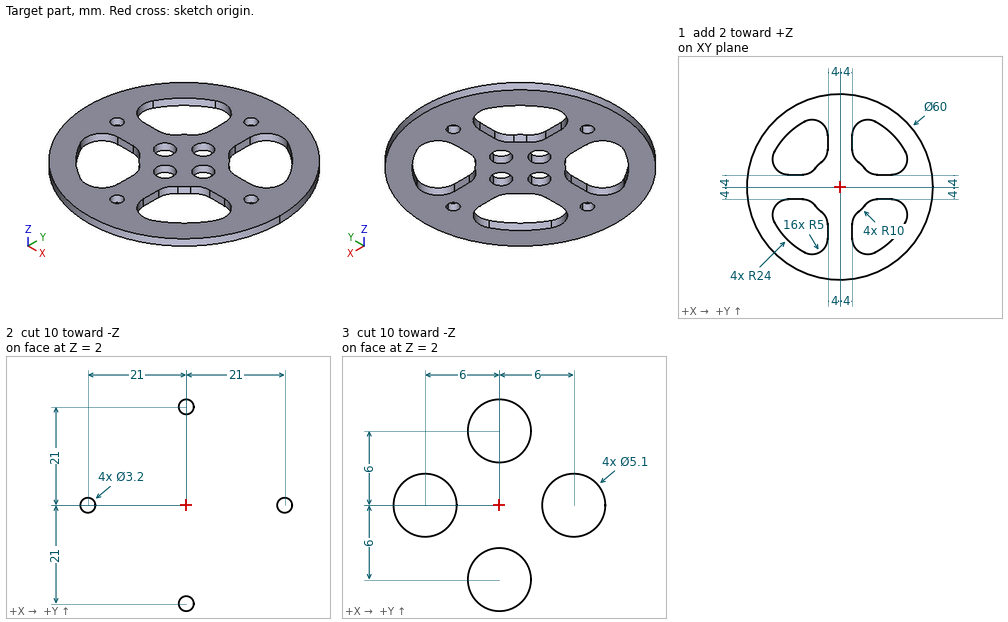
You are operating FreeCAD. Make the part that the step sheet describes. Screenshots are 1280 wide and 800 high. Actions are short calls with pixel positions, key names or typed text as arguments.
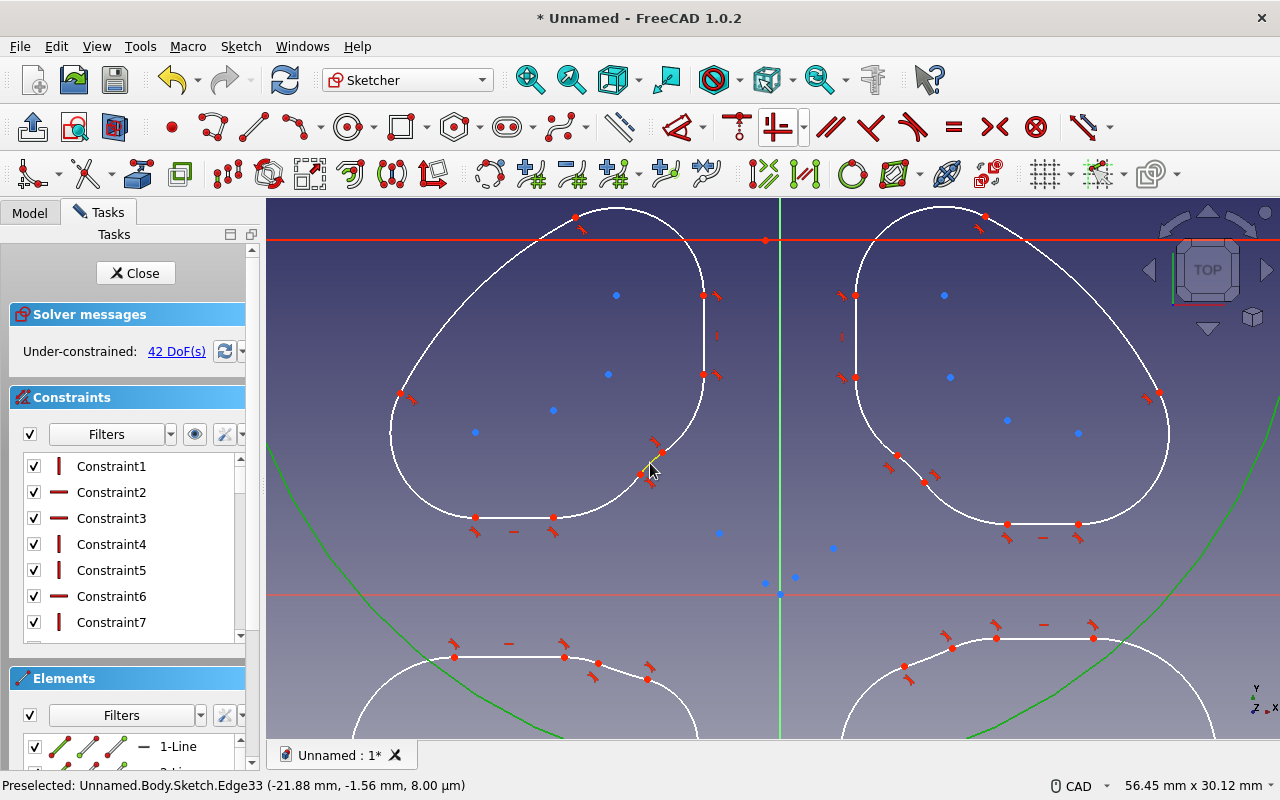
click(651, 463)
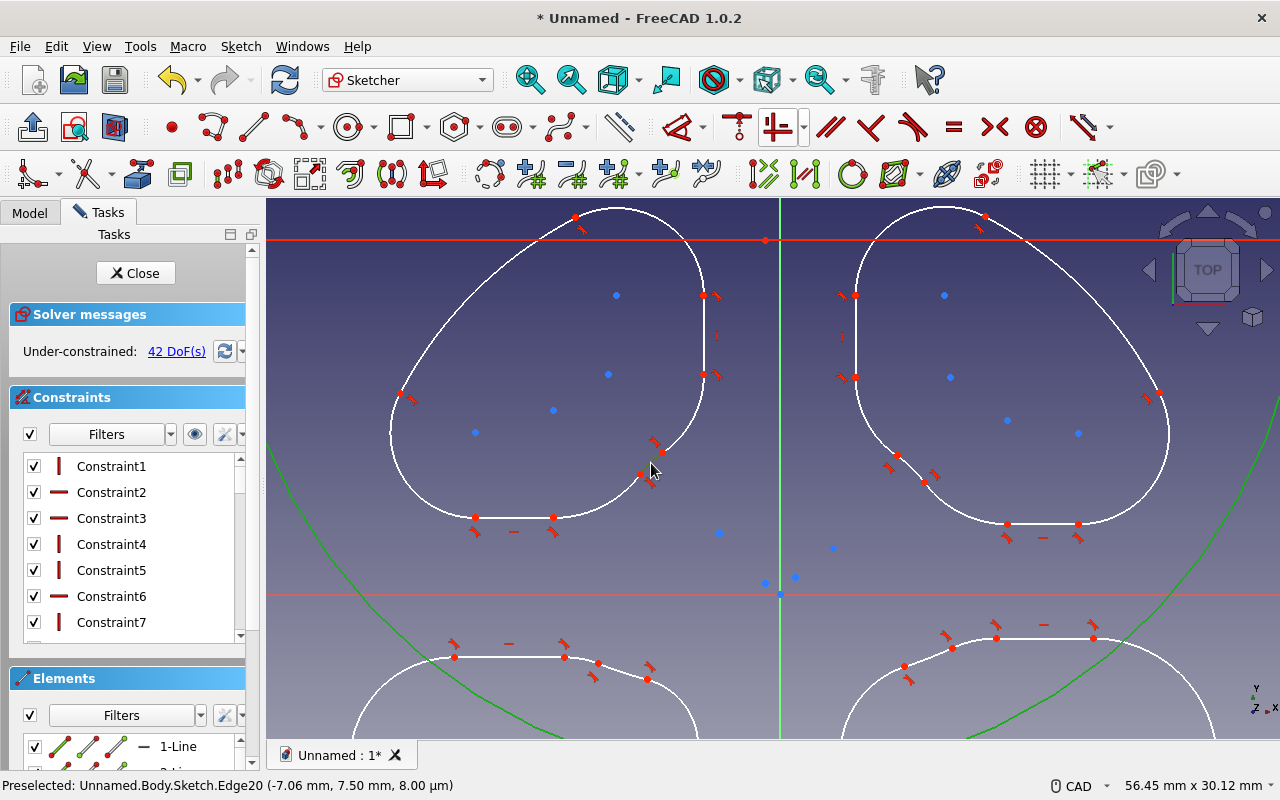
click(737, 128)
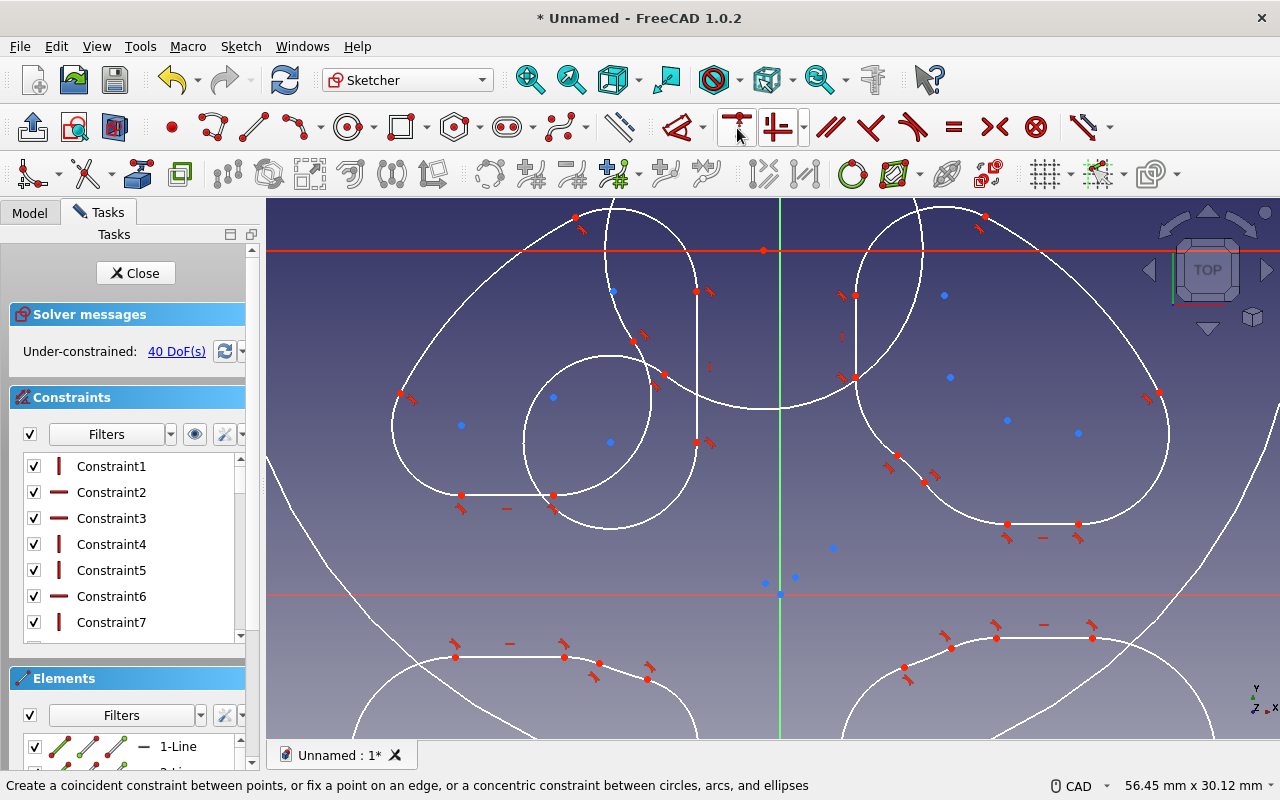
click(384, 633)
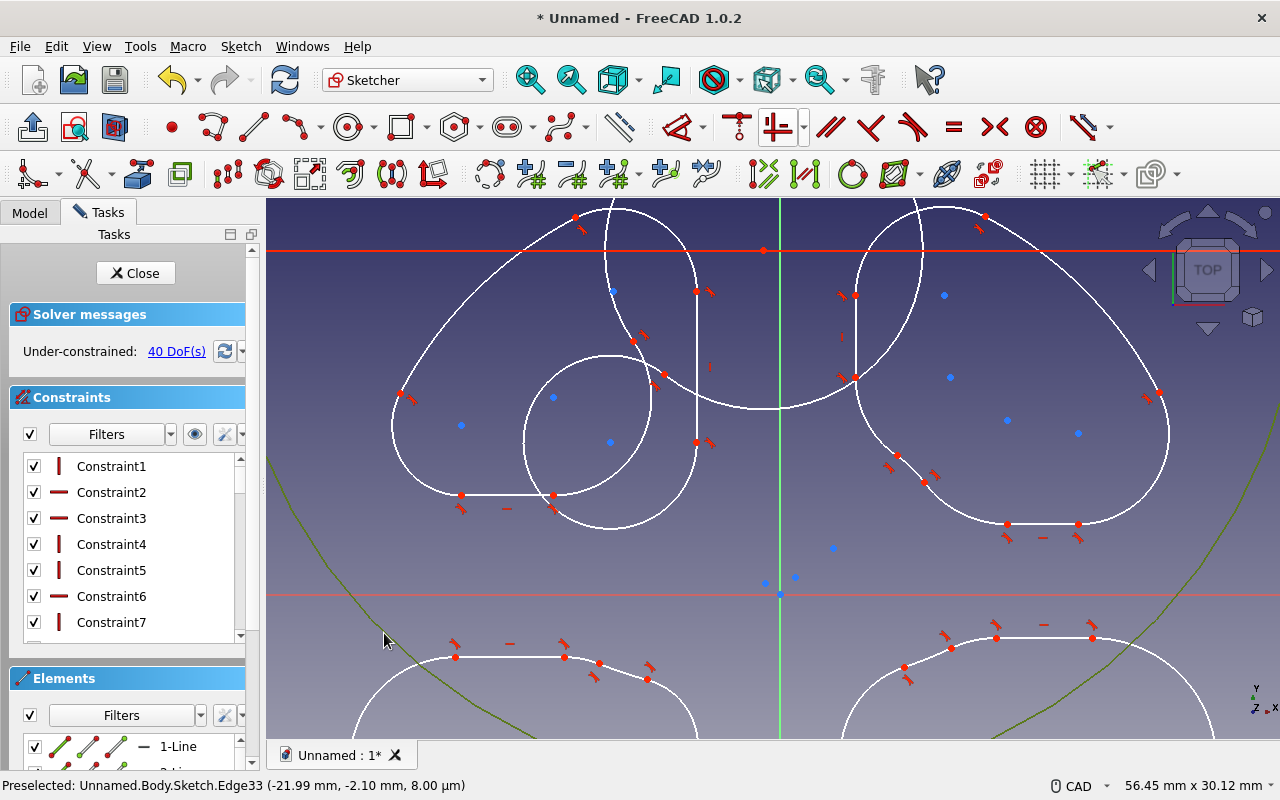
click(512, 259)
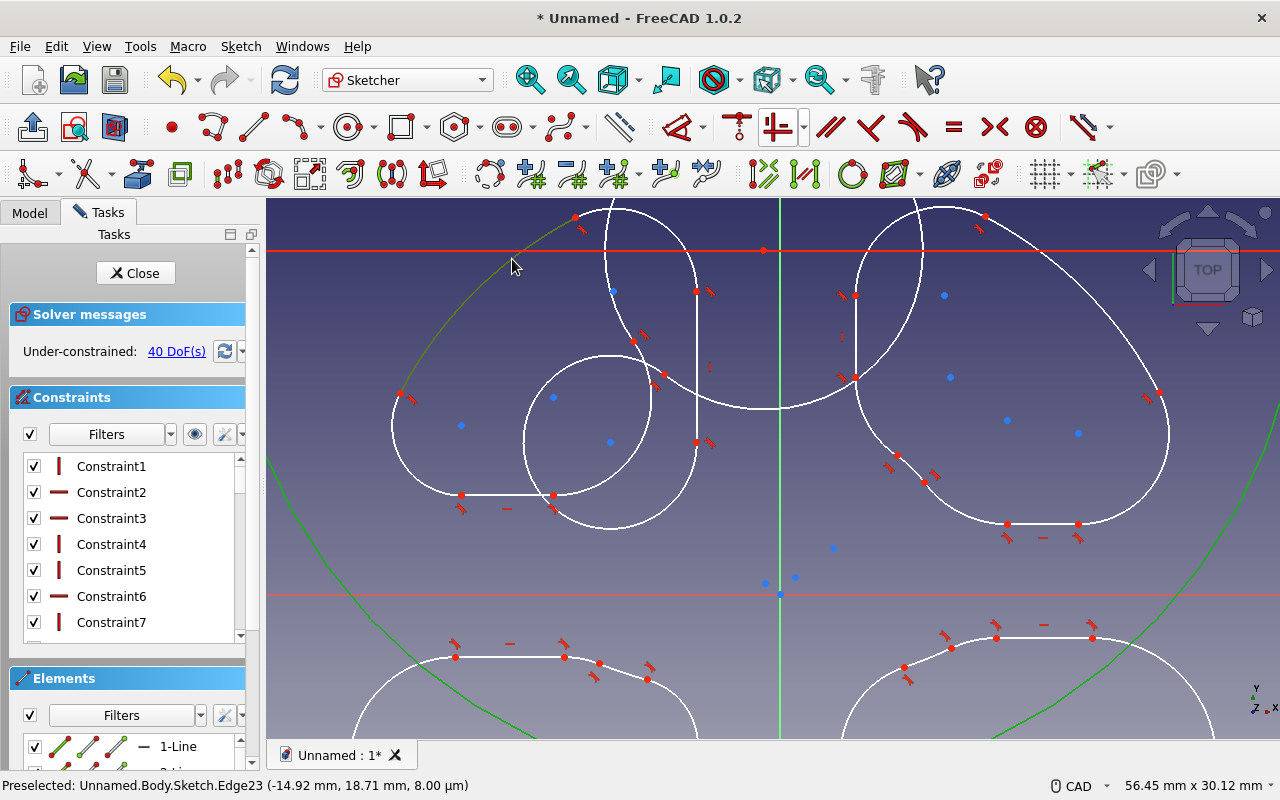
click(737, 128)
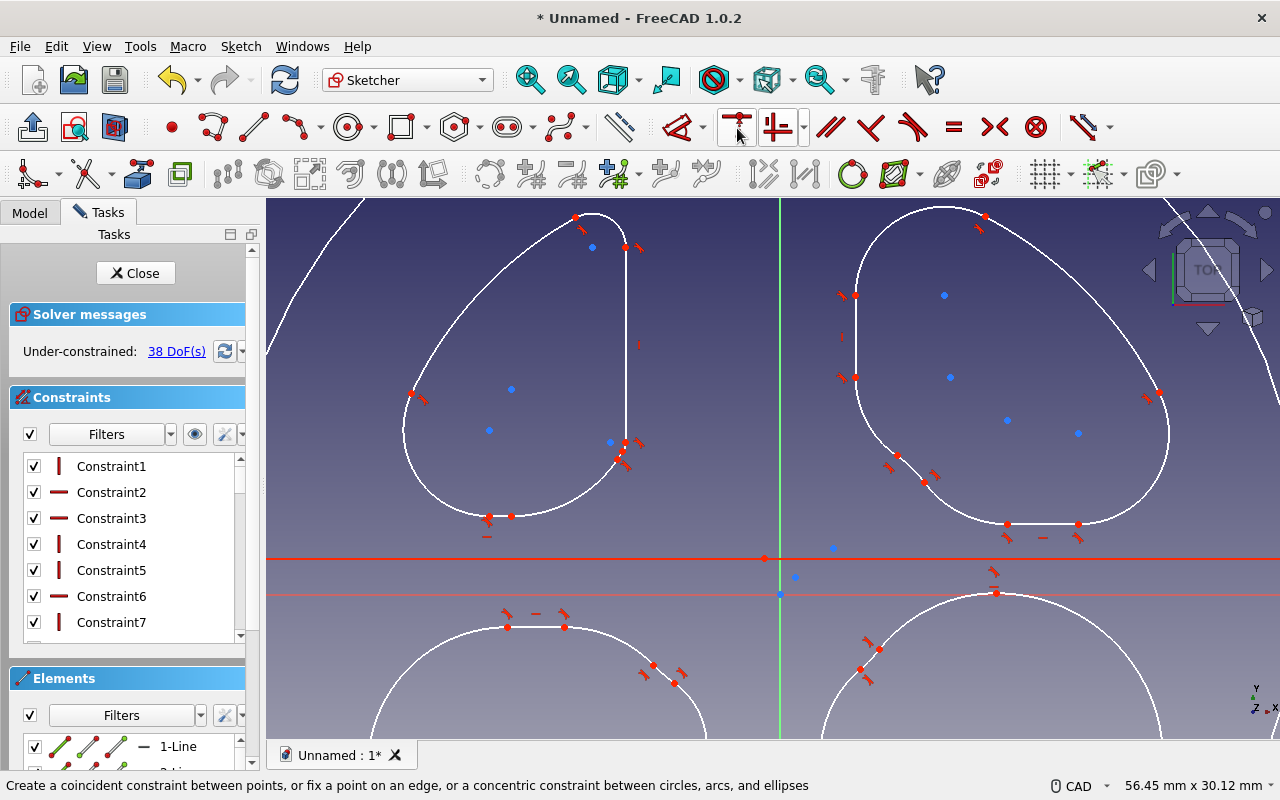
scroll(672, 414, down, 6)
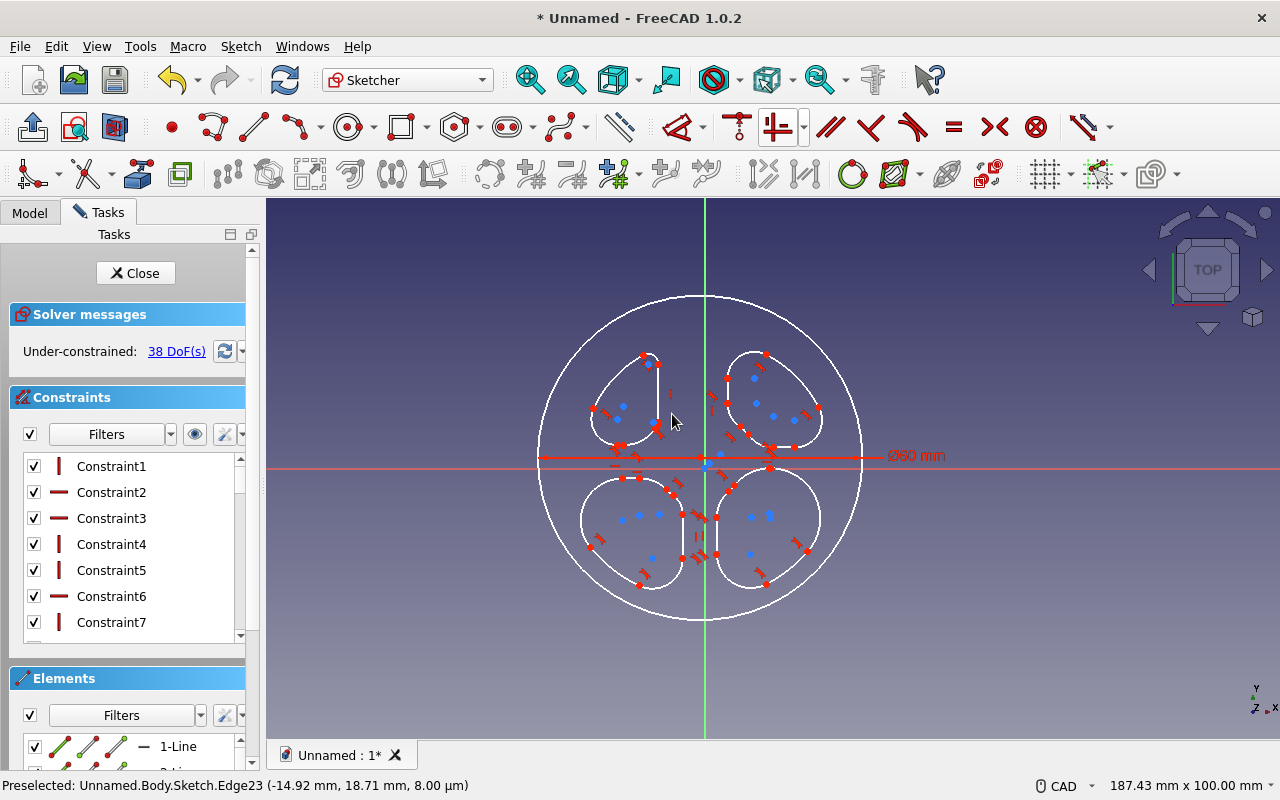
click(815, 343)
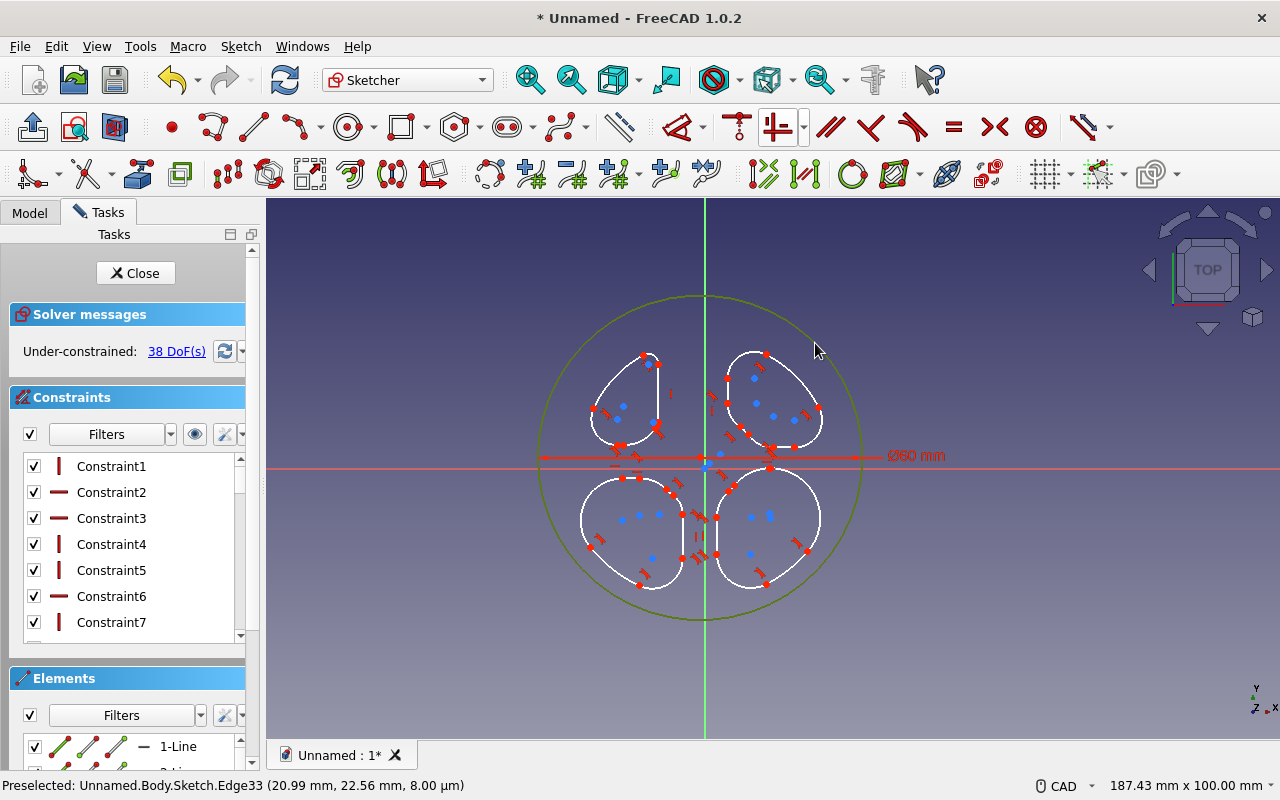
click(807, 389)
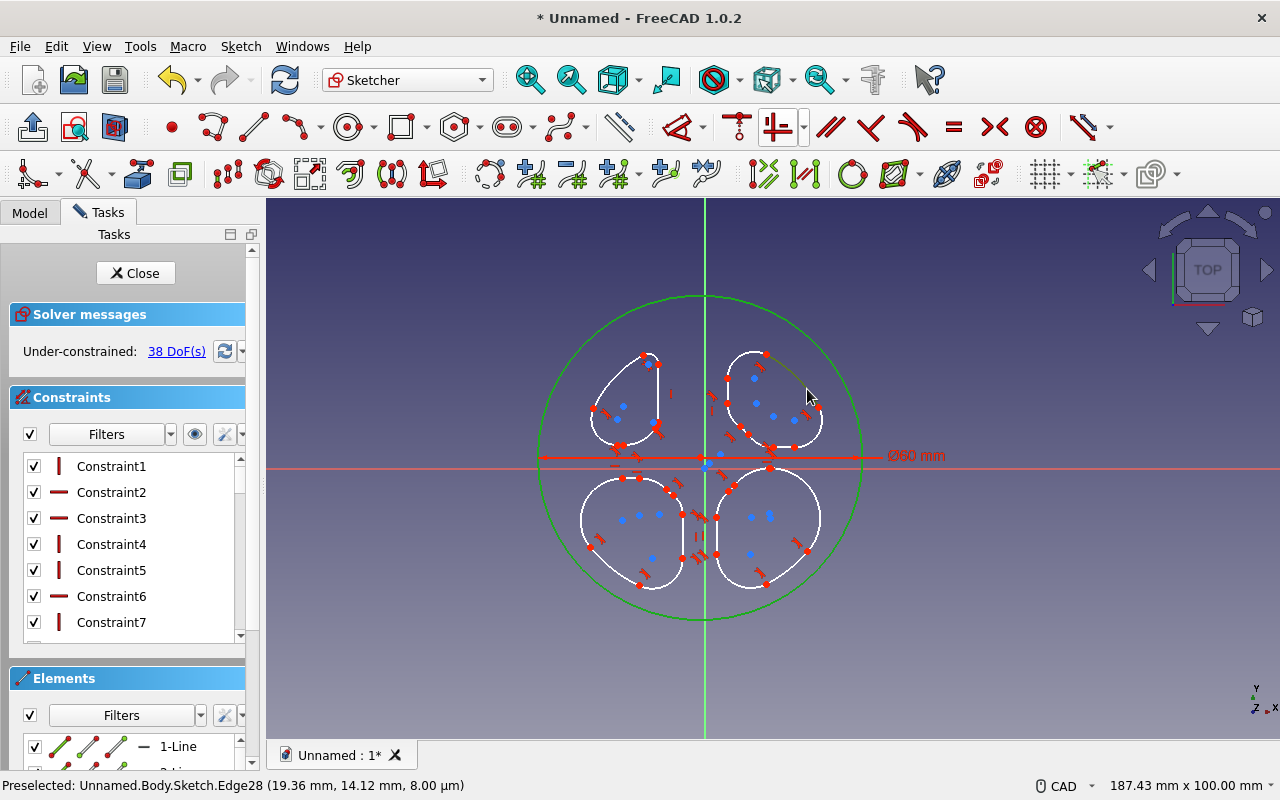
click(737, 128)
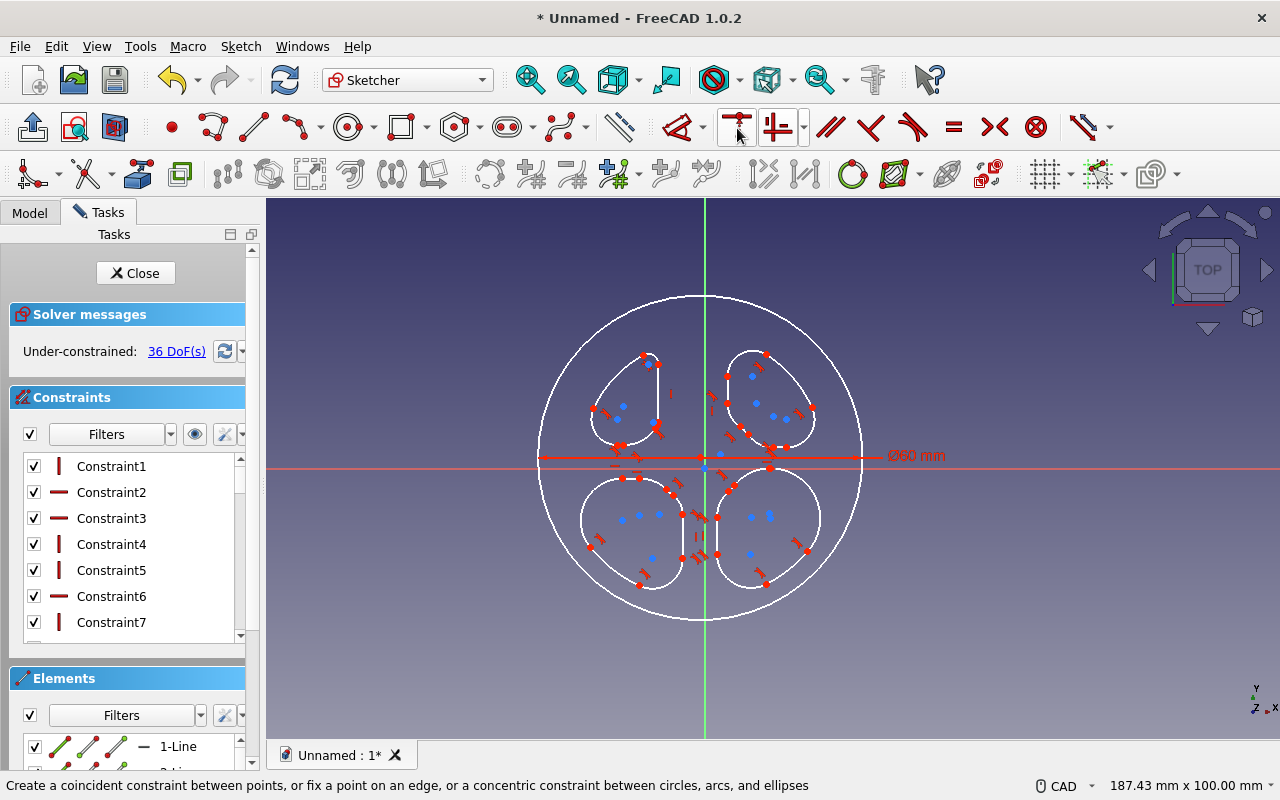
click(815, 343)